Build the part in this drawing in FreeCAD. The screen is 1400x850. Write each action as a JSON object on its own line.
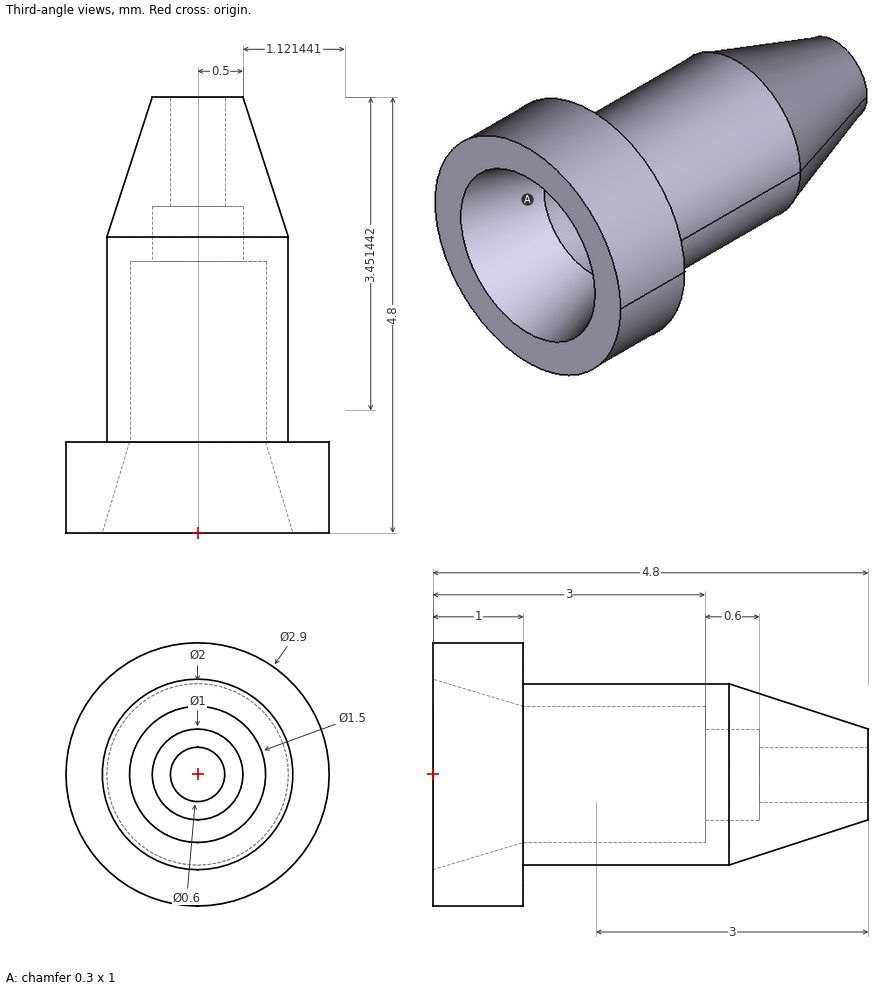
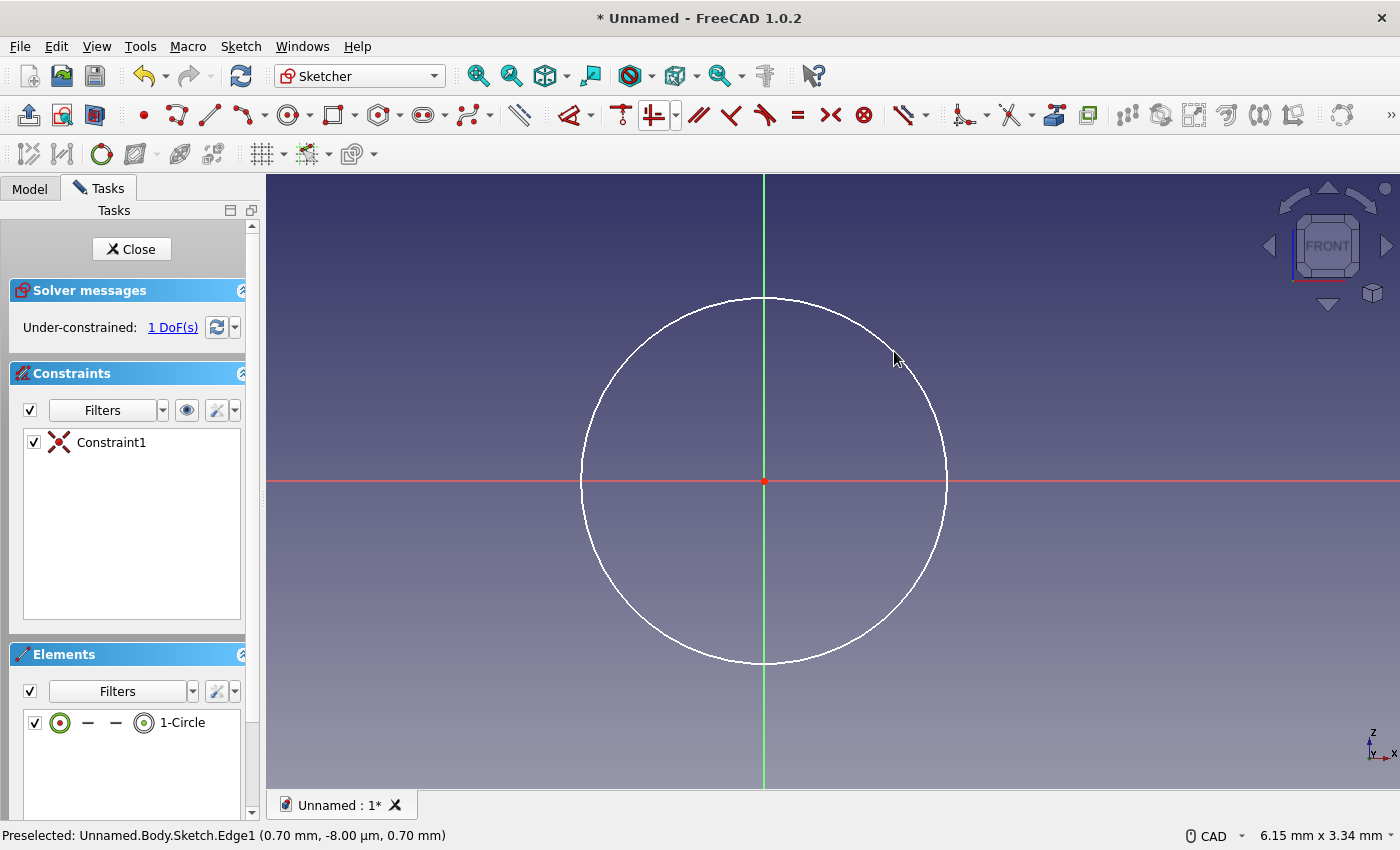
{"action": "left_click", "coordinate": [893, 351]}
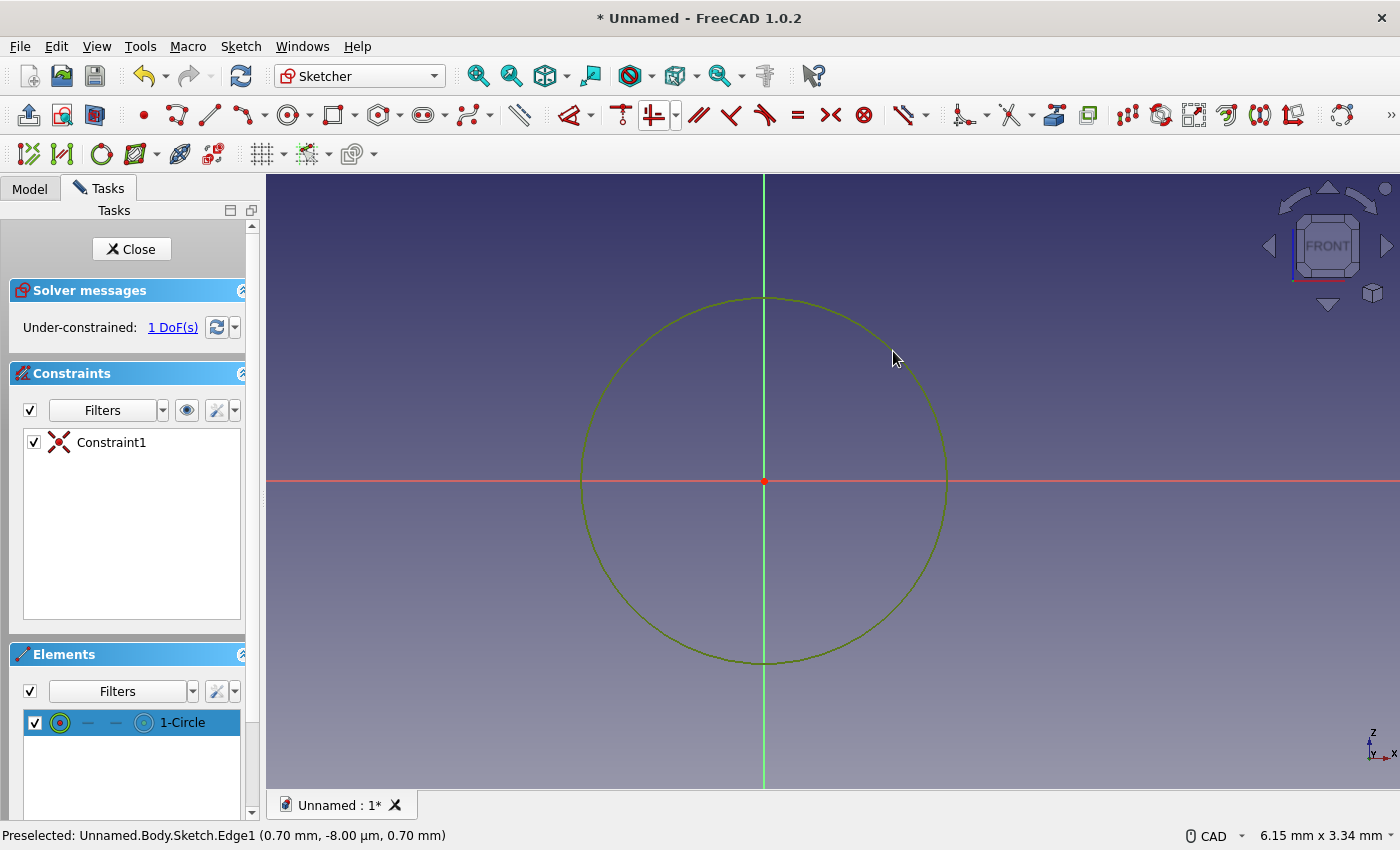
{"action": "left_click", "coordinate": [590, 116]}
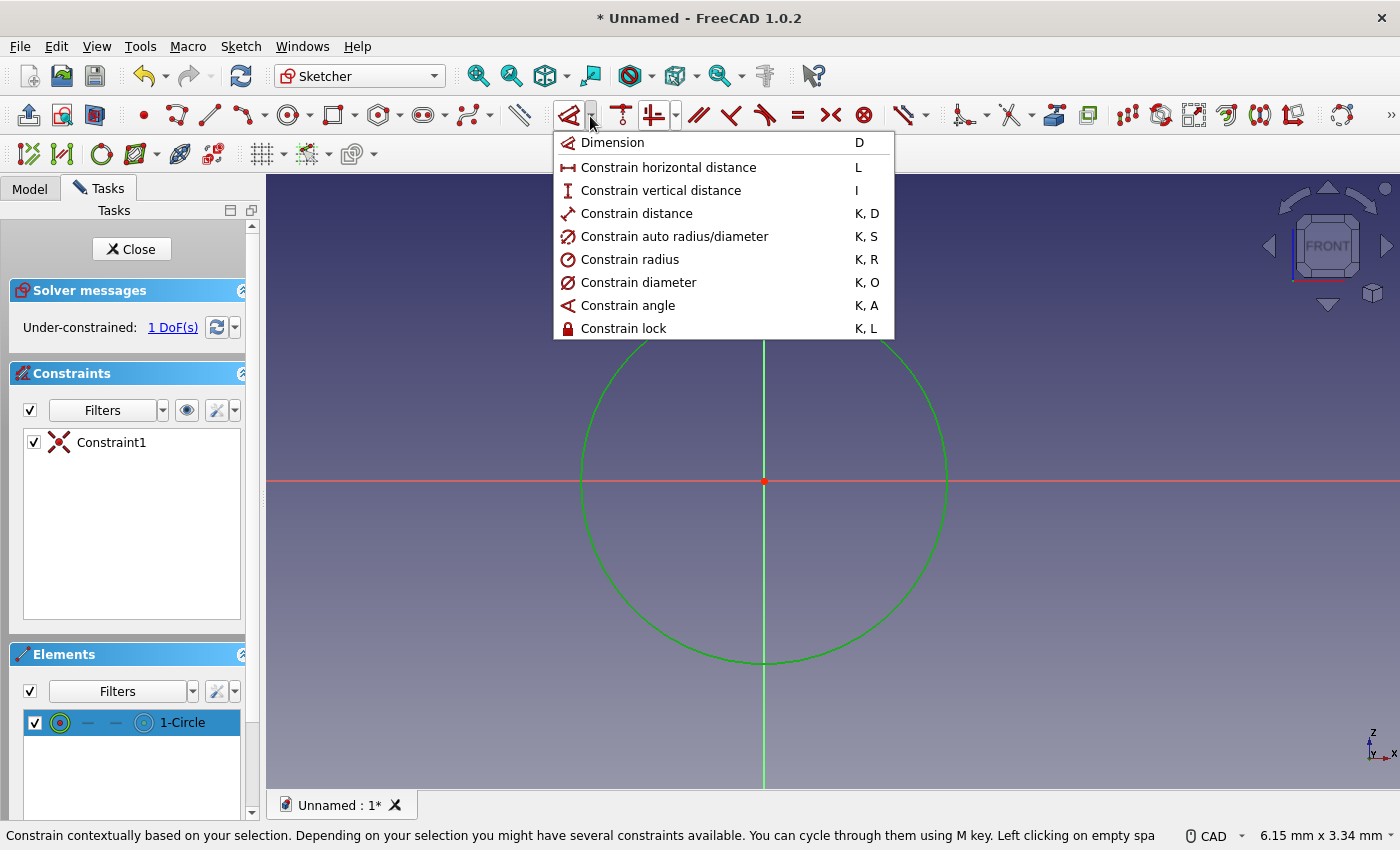
{"action": "left_click", "coordinate": [724, 282]}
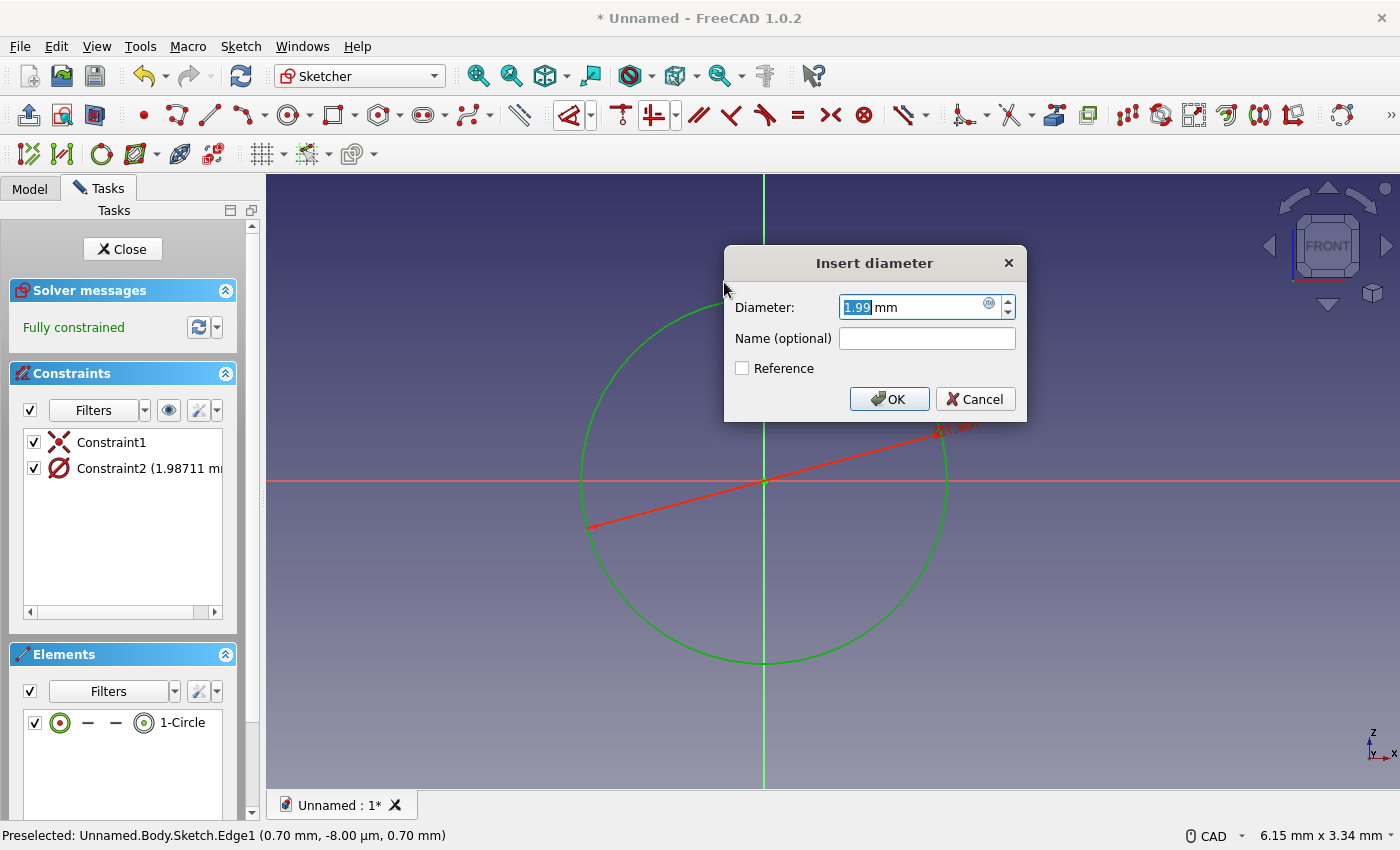
{"action": "type", "text": "2"}
{"action": "key", "text": "Return"}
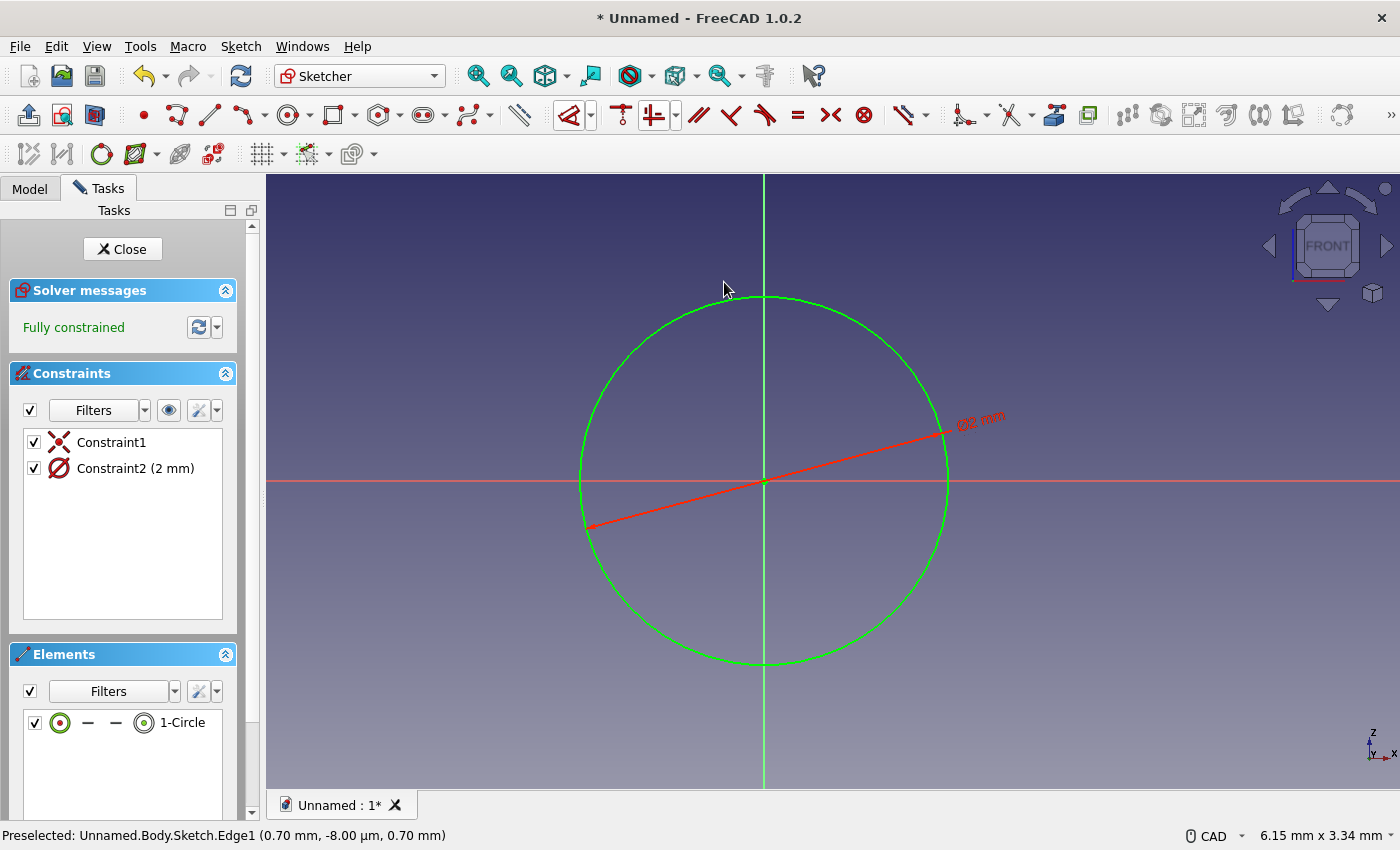
{"action": "left_click", "coordinate": [123, 249]}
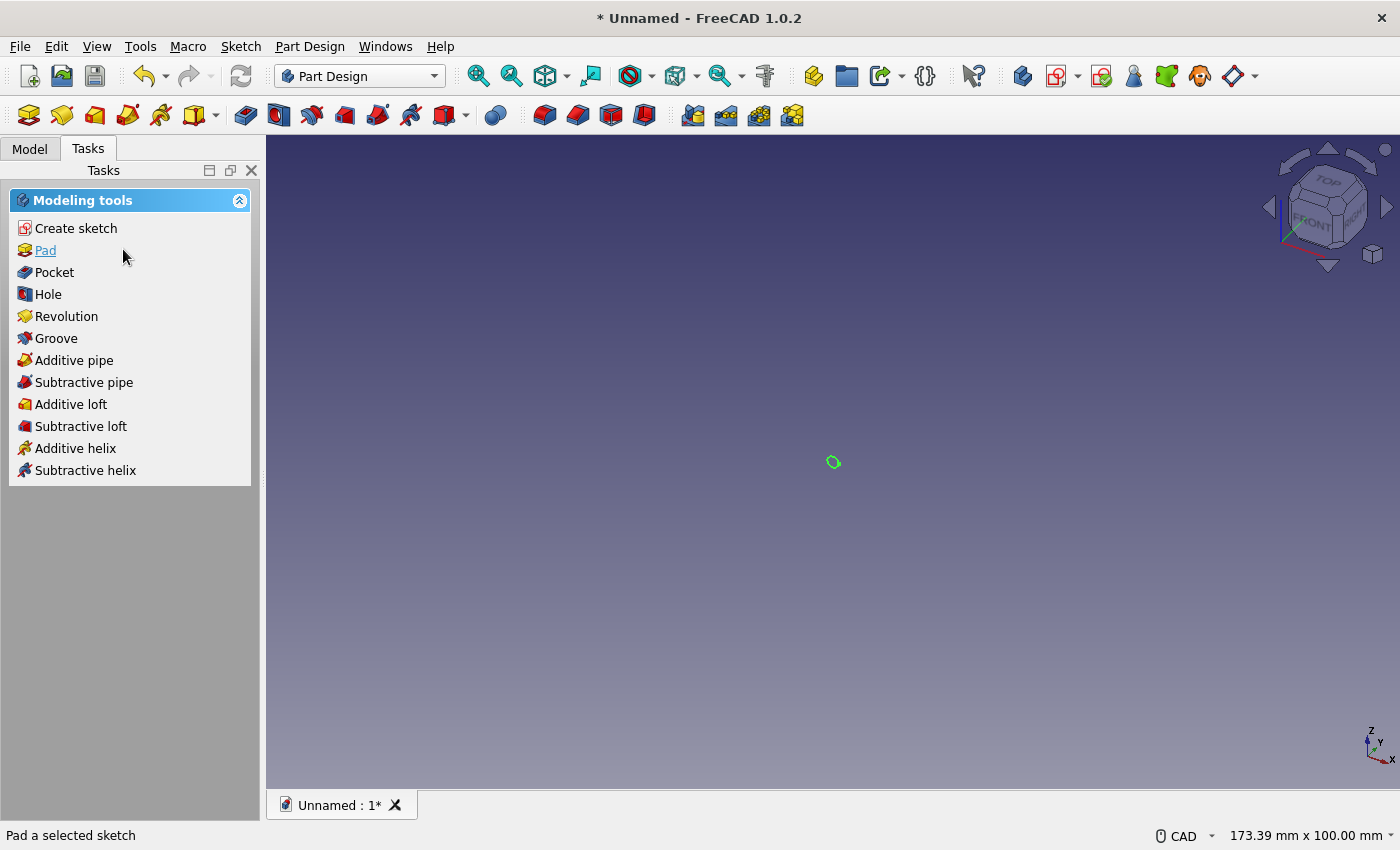
{"action": "left_click", "coordinate": [29, 116]}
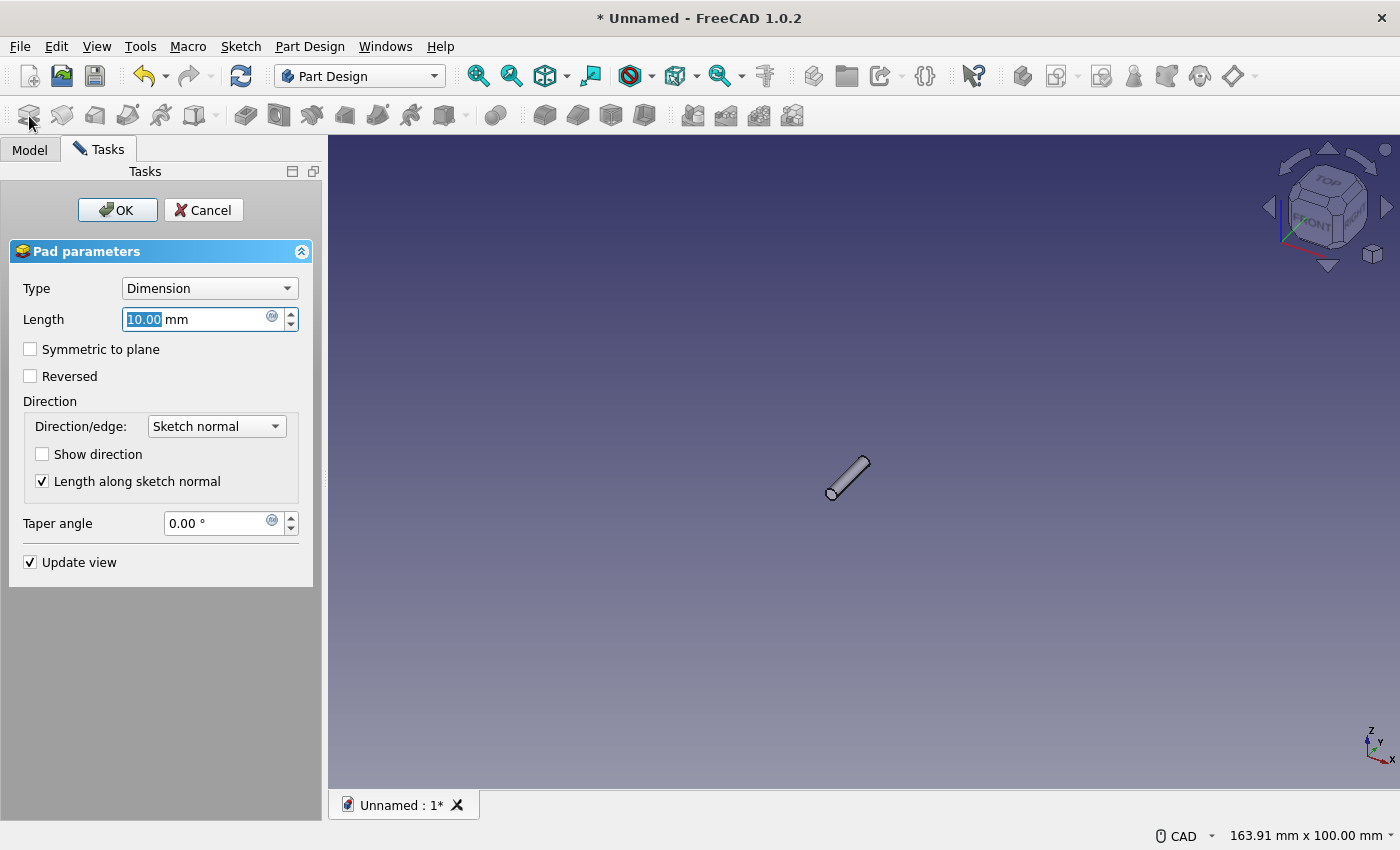
{"action": "type", "text": "4.8"}
{"action": "key", "text": "Tab"}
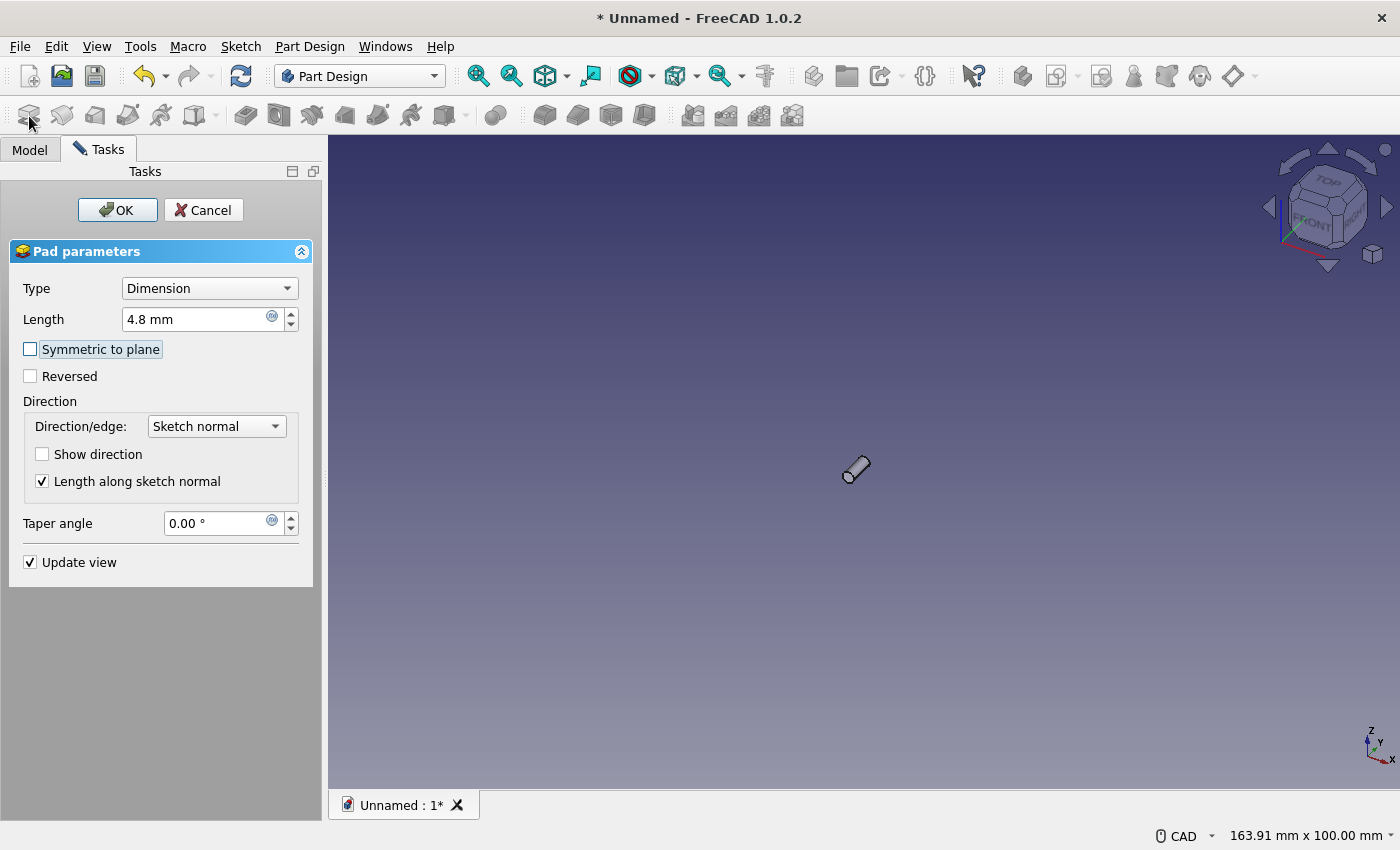
{"action": "left_click", "coordinate": [31, 376]}